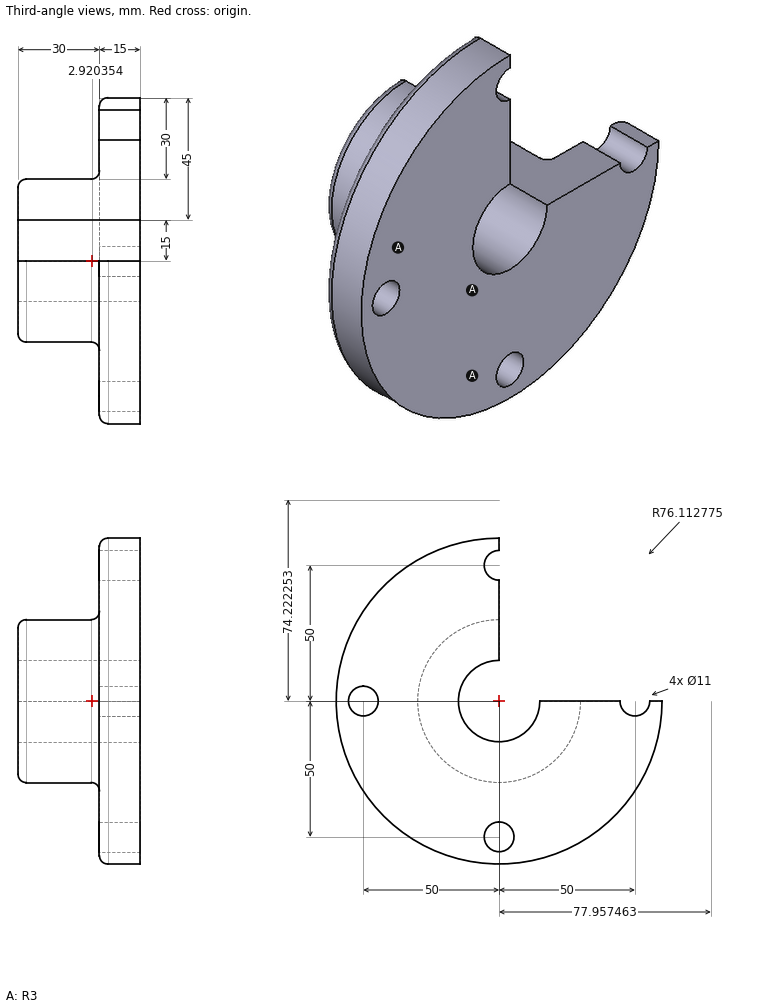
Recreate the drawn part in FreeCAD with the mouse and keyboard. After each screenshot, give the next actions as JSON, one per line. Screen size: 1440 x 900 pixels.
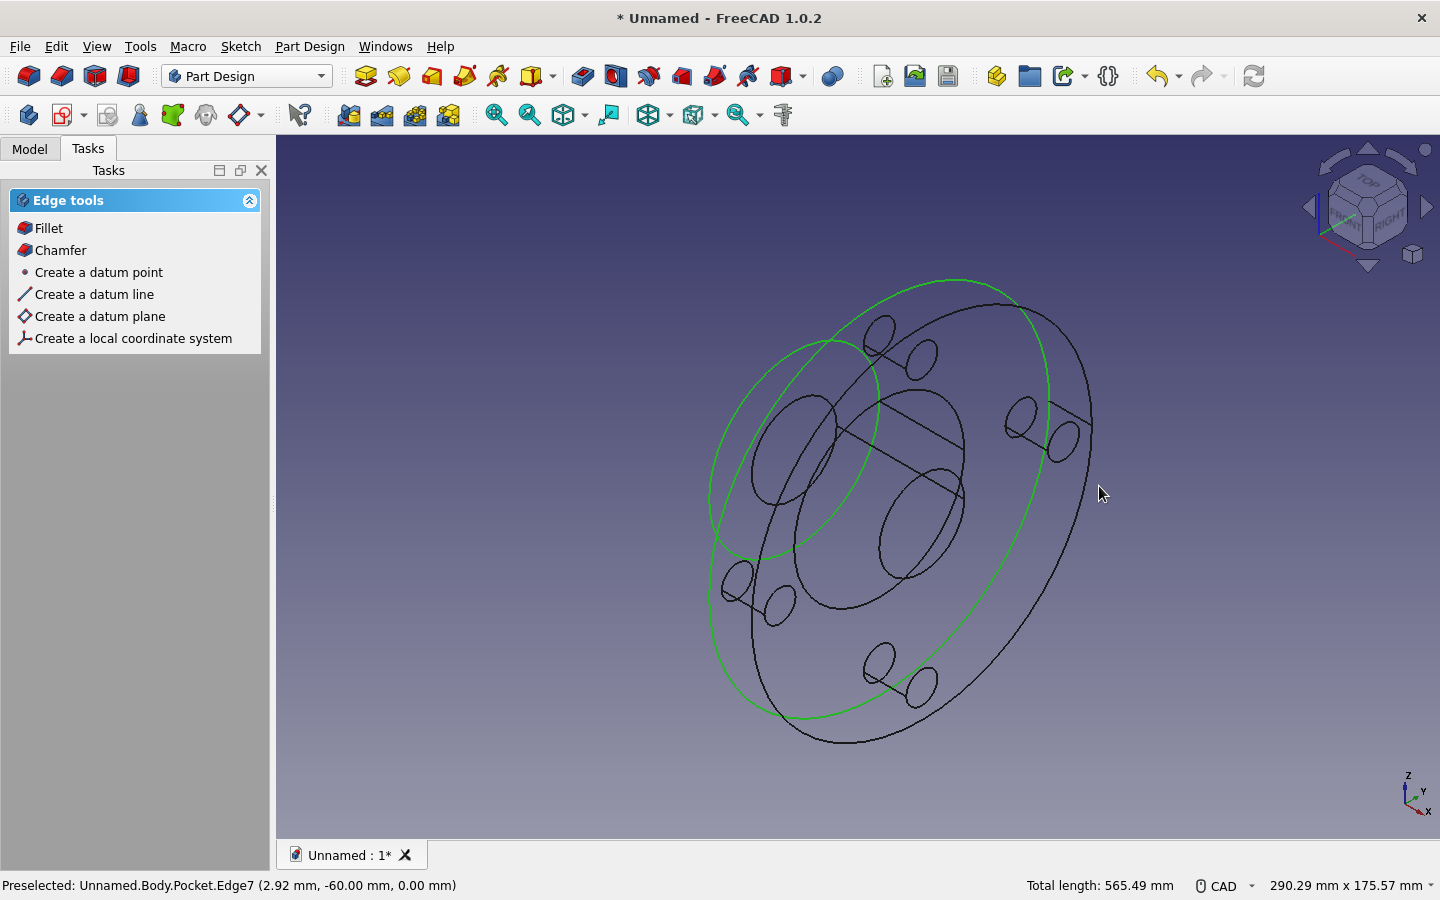
{"action": "left_click", "coordinate": [794, 547], "text": "ctrl"}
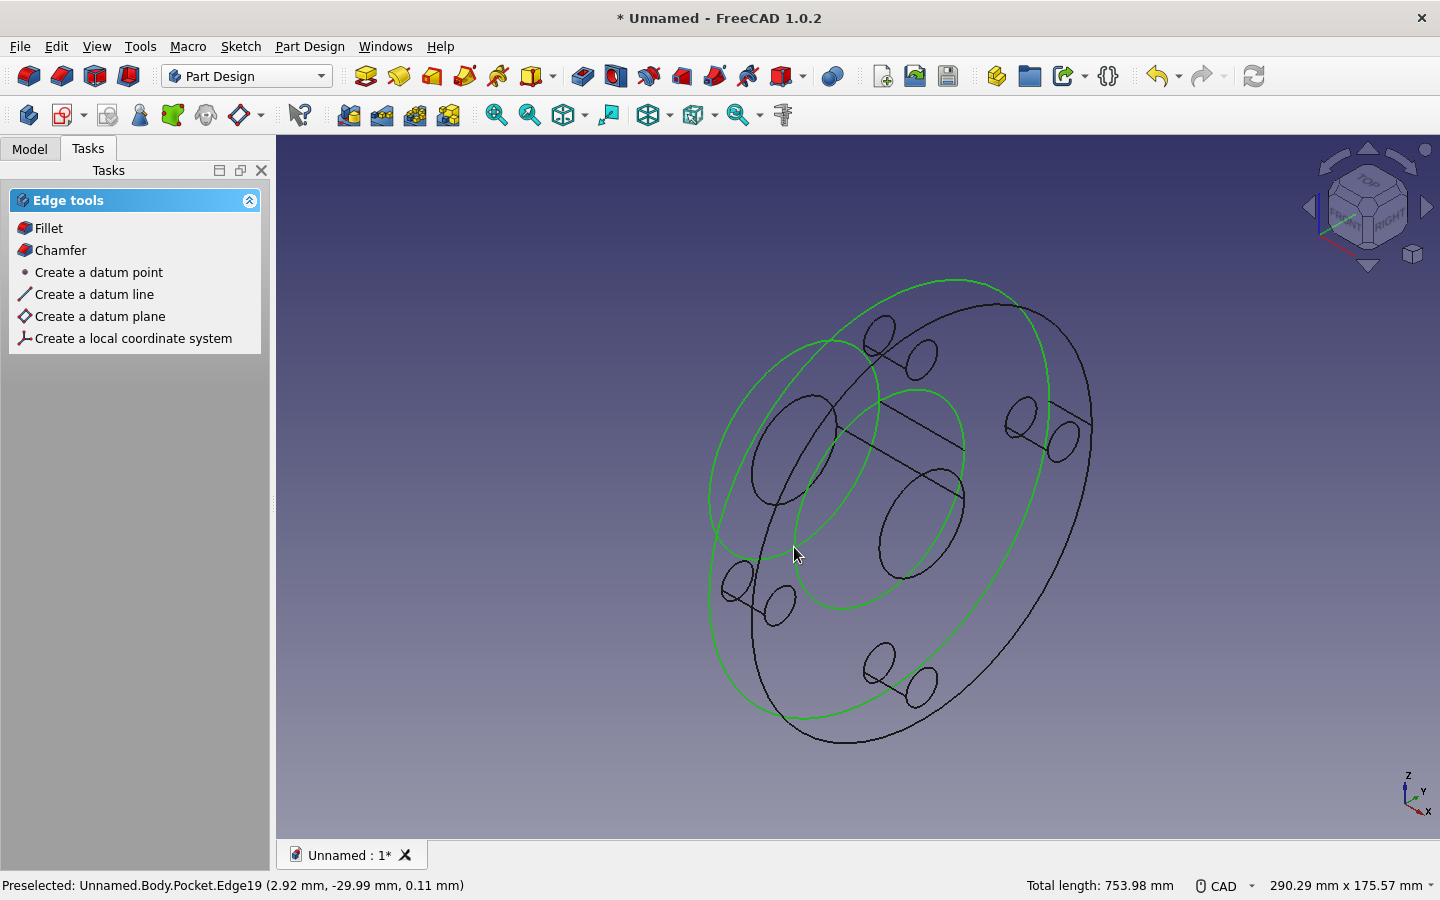
{"action": "key", "text": "v 1"}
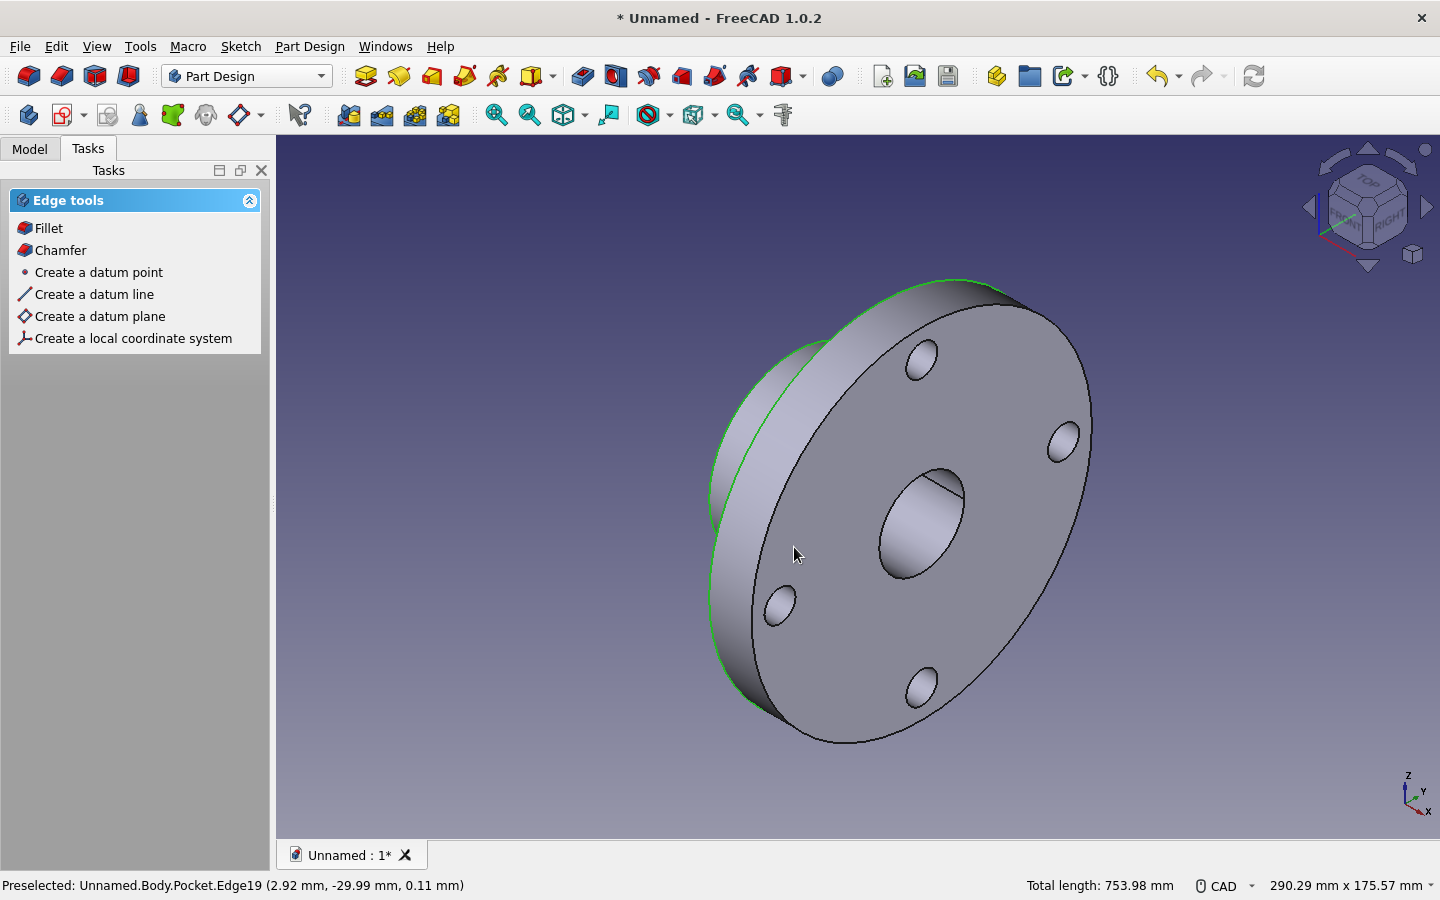
{"action": "left_click", "coordinate": [29, 76]}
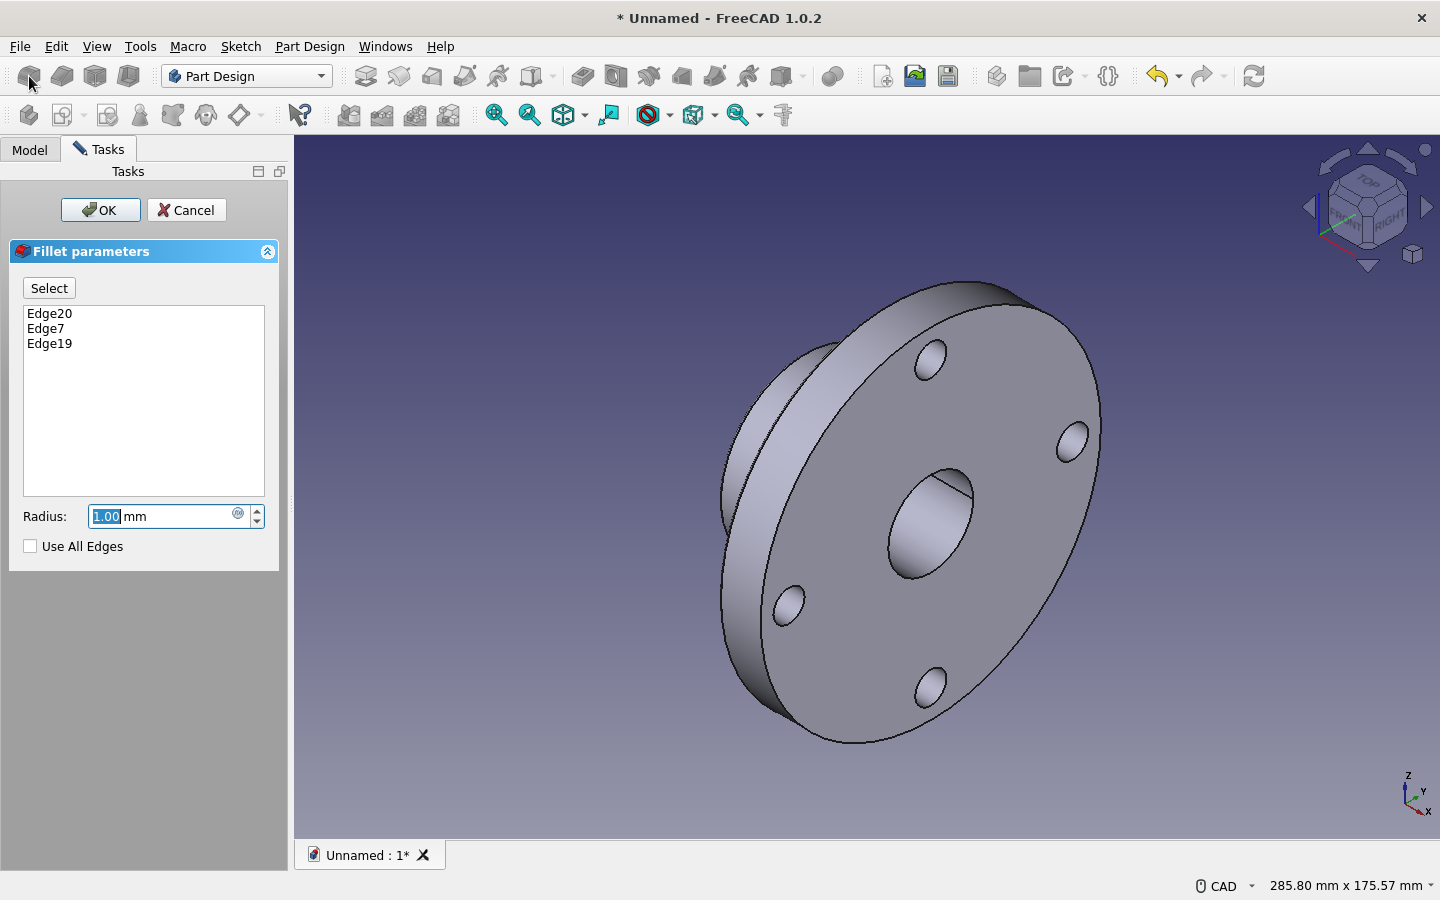
{"action": "type", "text": "3"}
{"action": "key", "text": "Tab"}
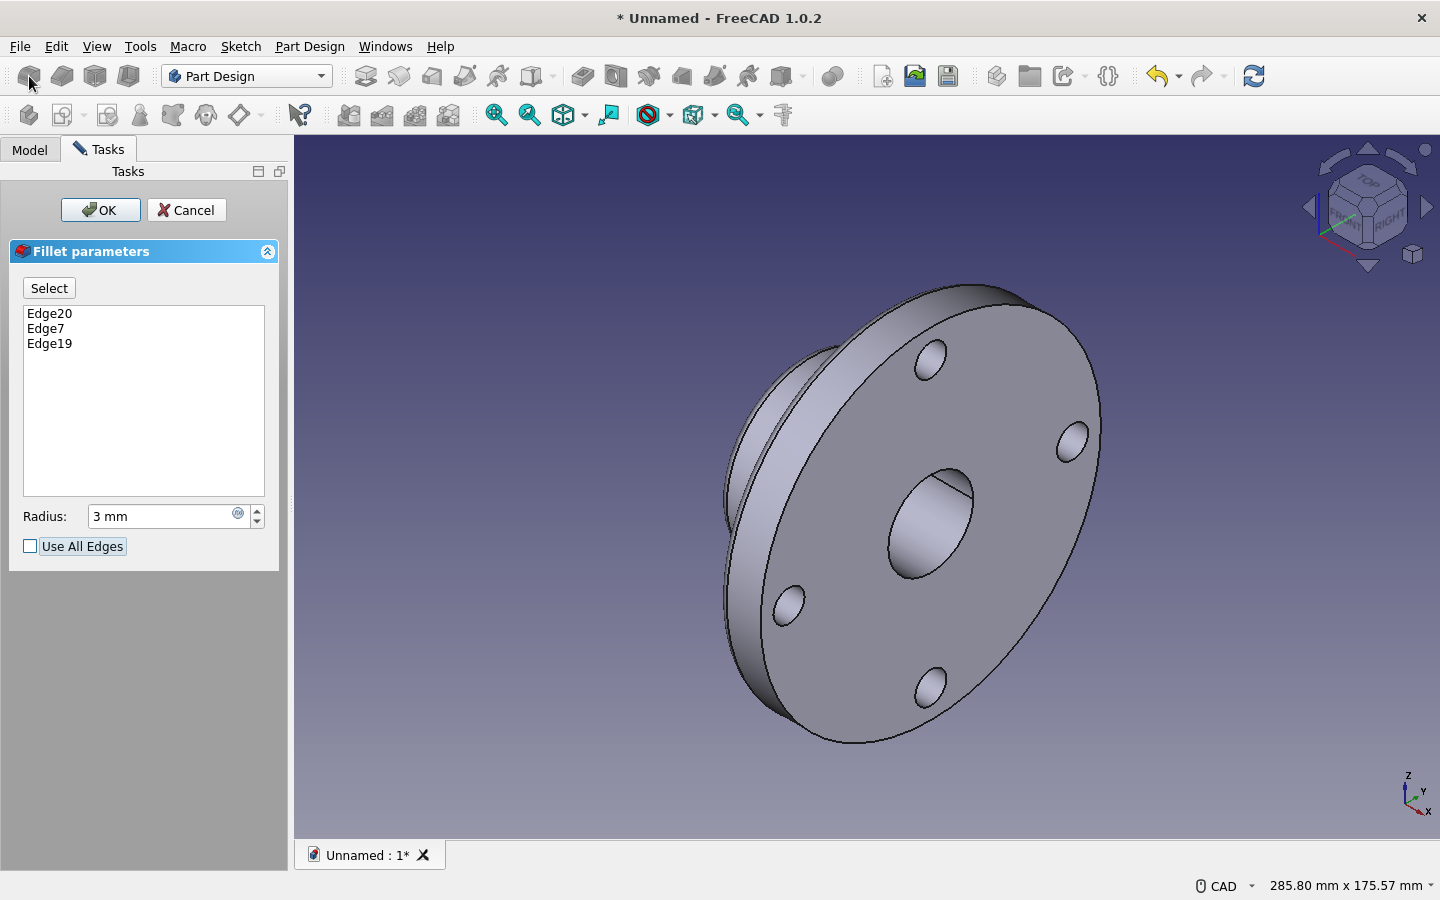
{"action": "left_click", "coordinate": [101, 210]}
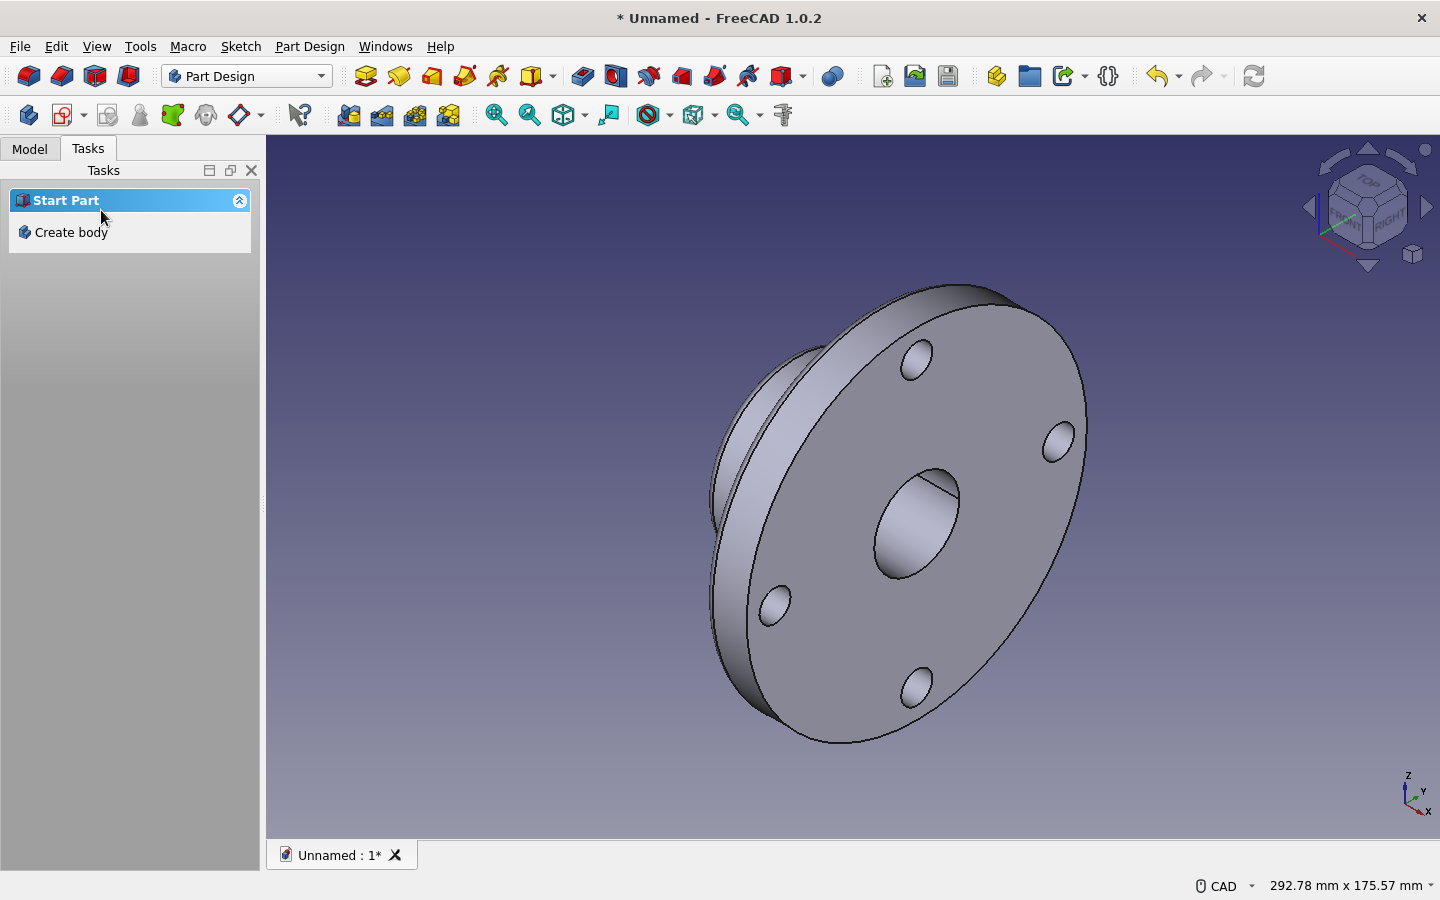
{"action": "key", "text": "6"}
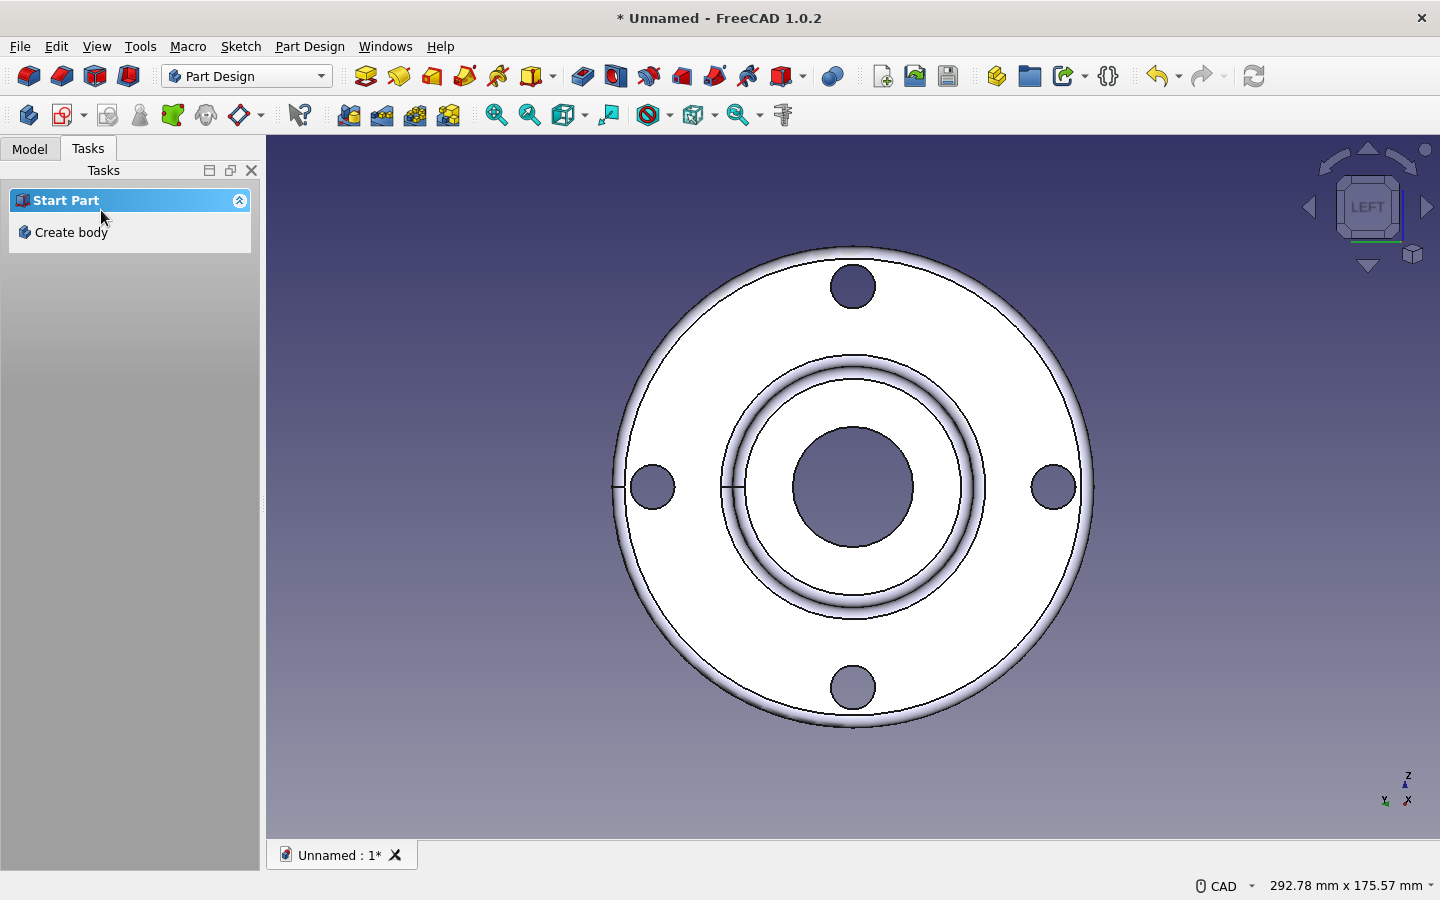
{"action": "left_click", "coordinate": [915, 548]}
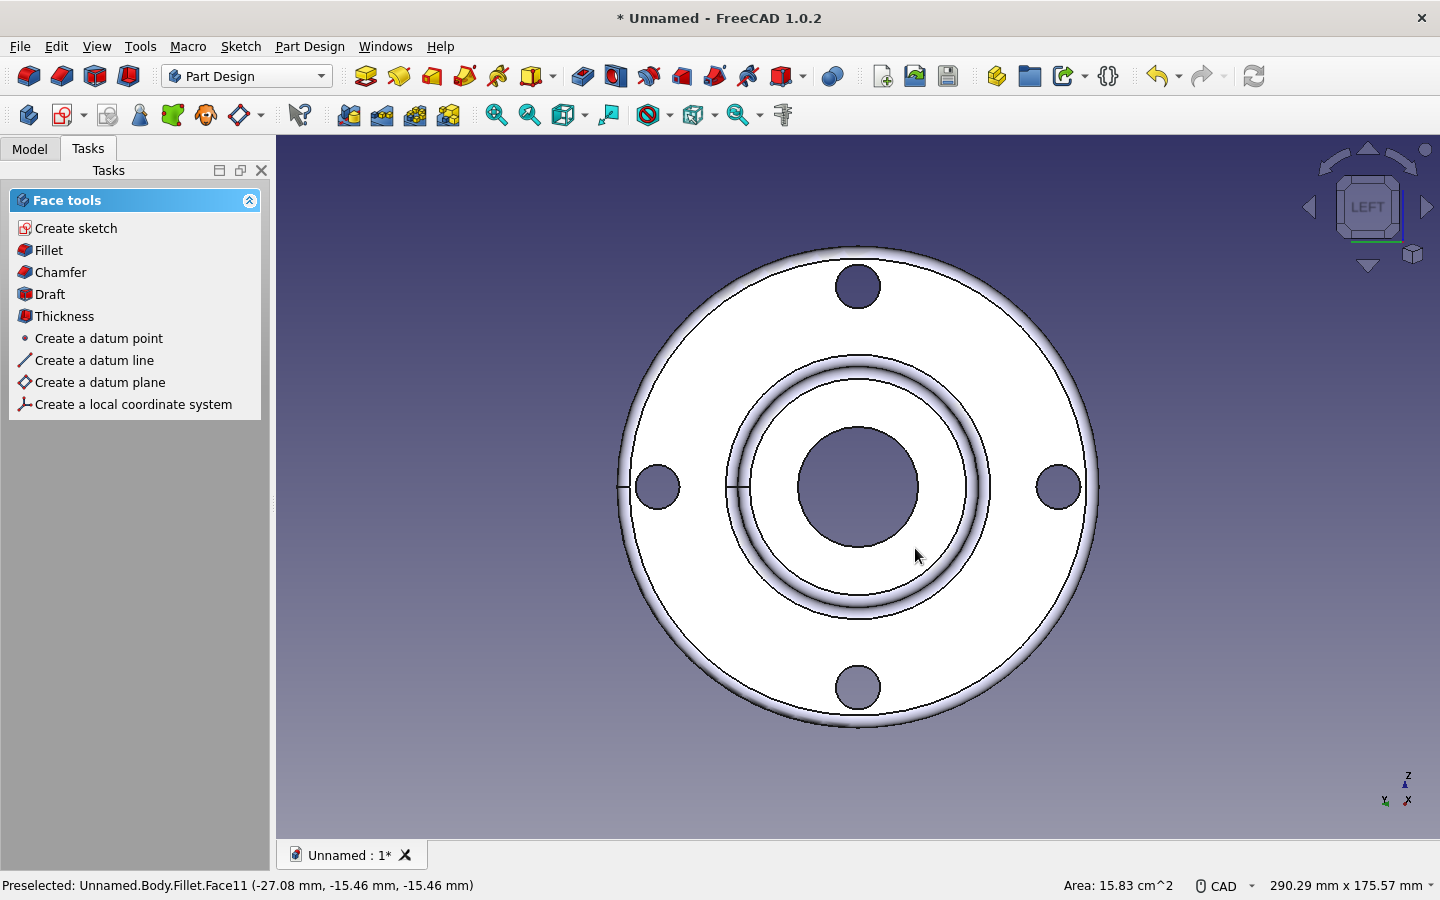
{"action": "left_click", "coordinate": [62, 116]}